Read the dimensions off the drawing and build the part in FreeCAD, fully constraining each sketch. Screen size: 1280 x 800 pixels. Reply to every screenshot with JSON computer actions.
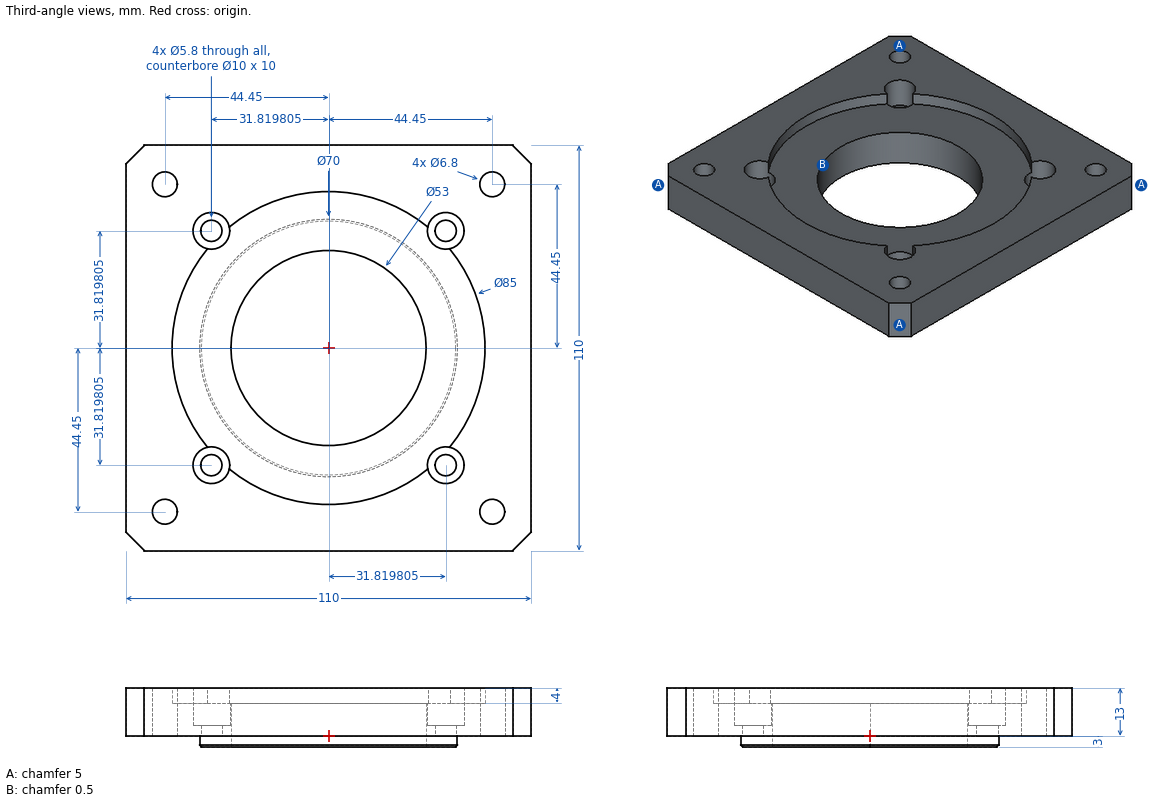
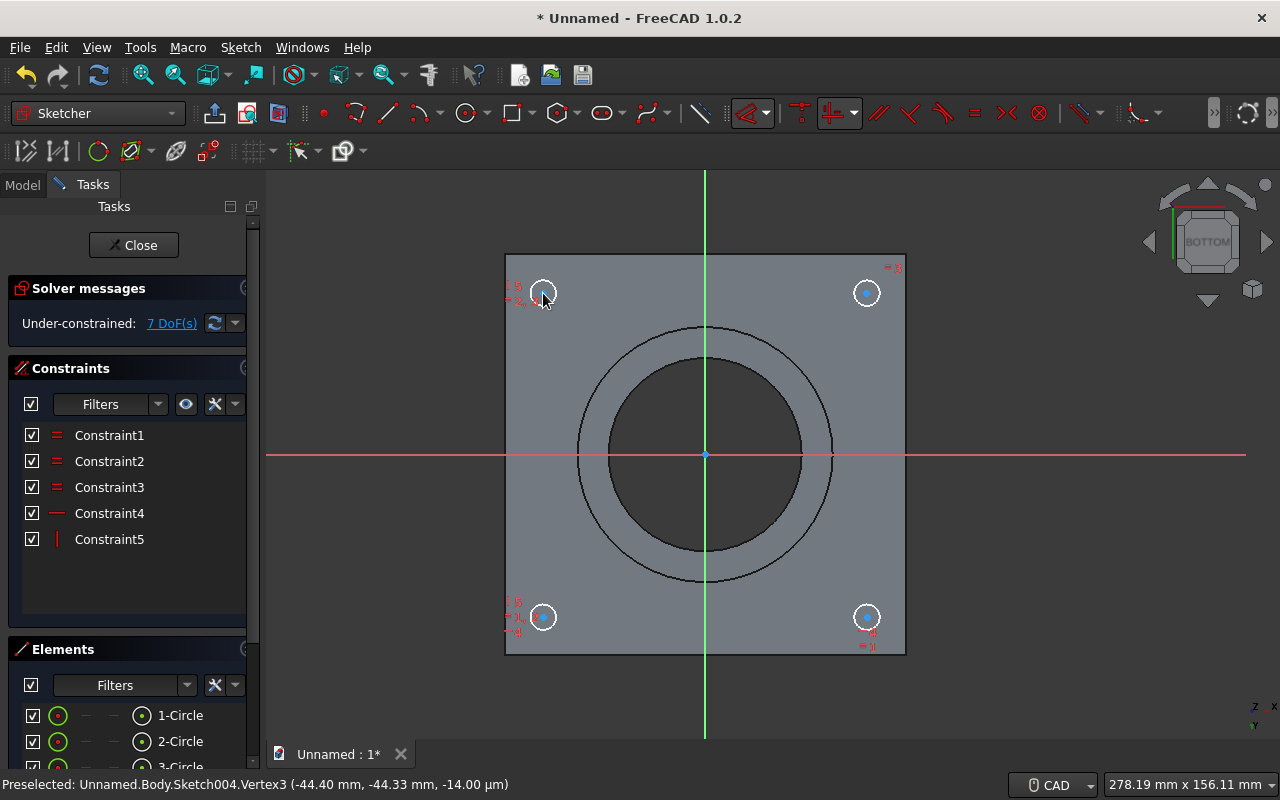
{"action": "left_click", "coordinate": [867, 617]}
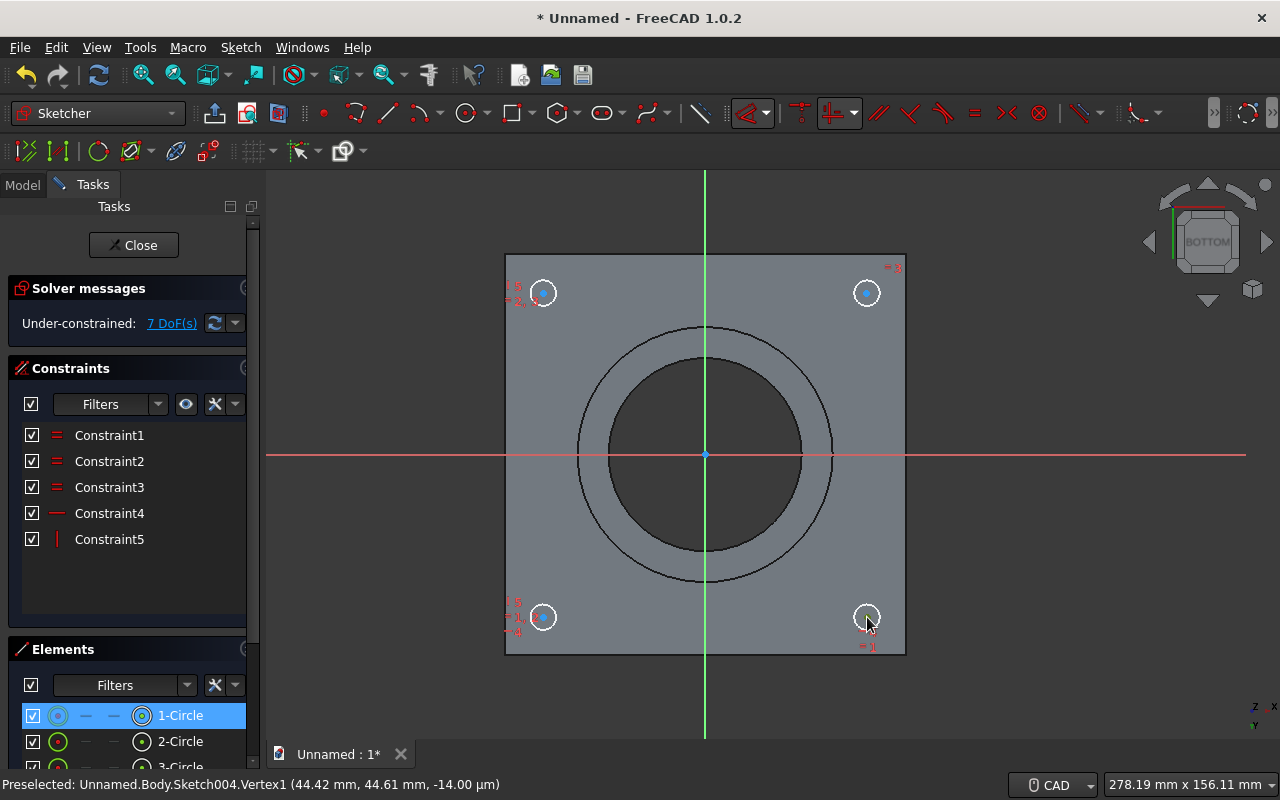
{"action": "left_click", "coordinate": [867, 293]}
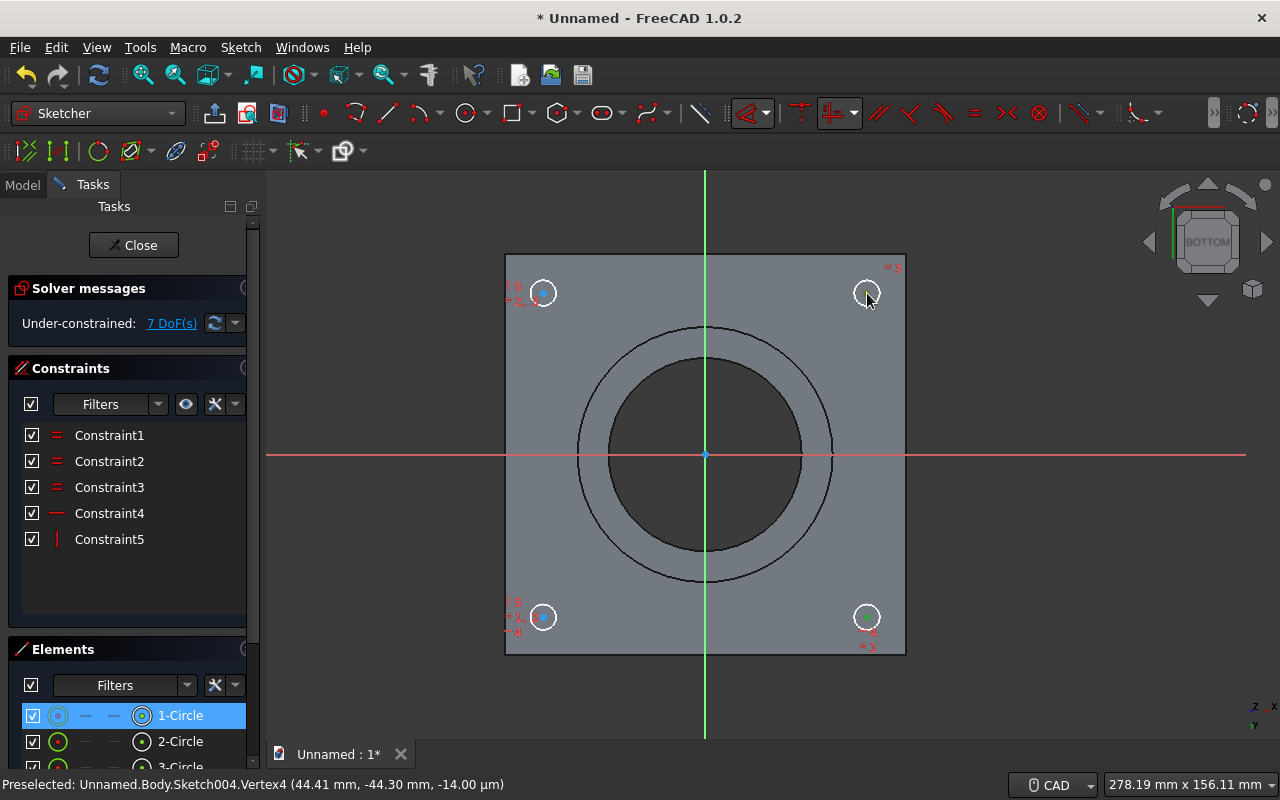
{"action": "key", "text": "v"}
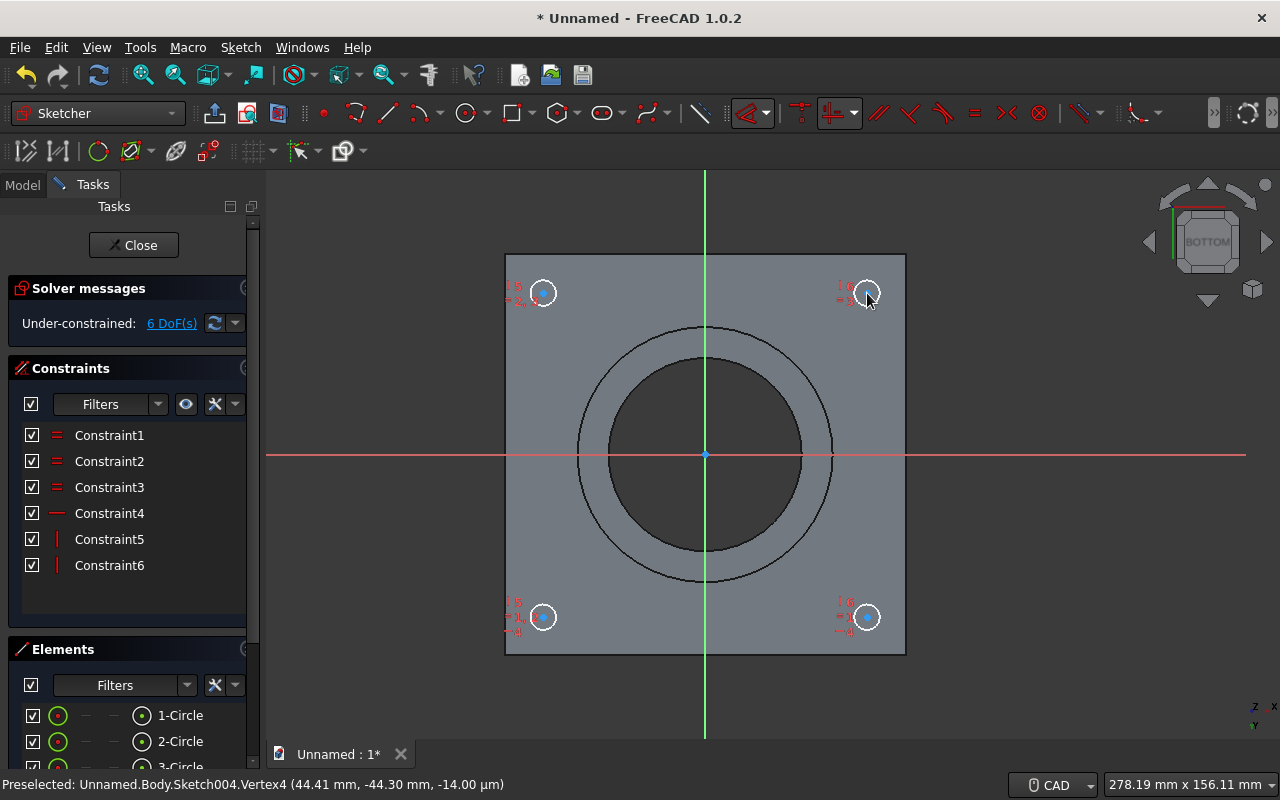
{"action": "left_click", "coordinate": [543, 293]}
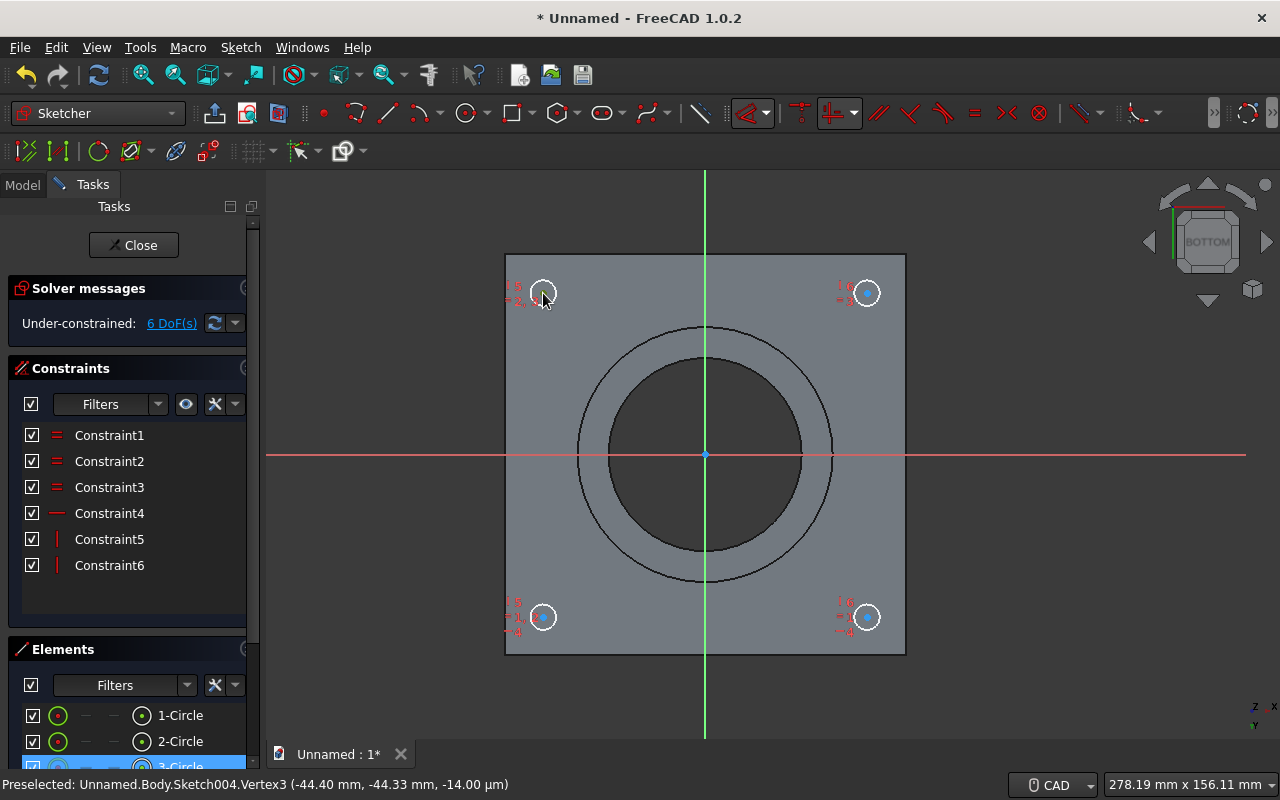
{"action": "left_click", "coordinate": [867, 293]}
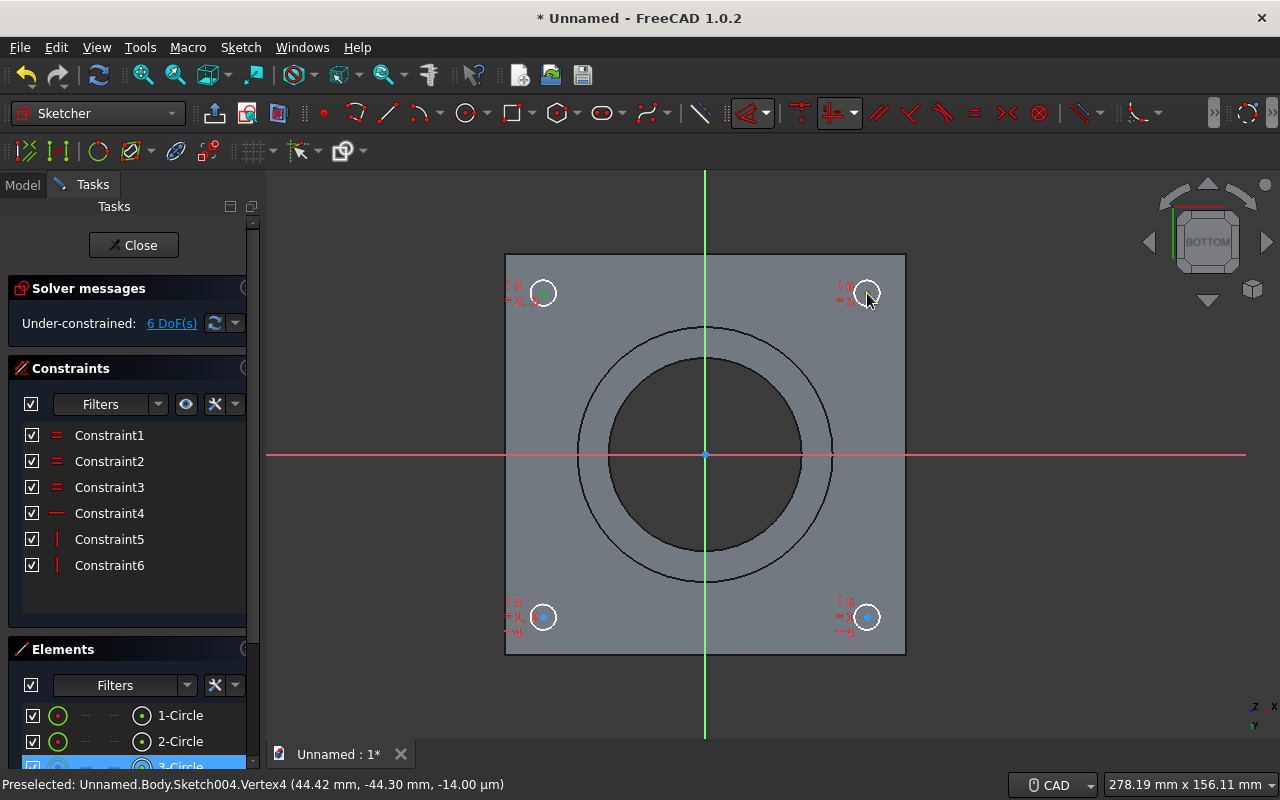
{"action": "key", "text": "h"}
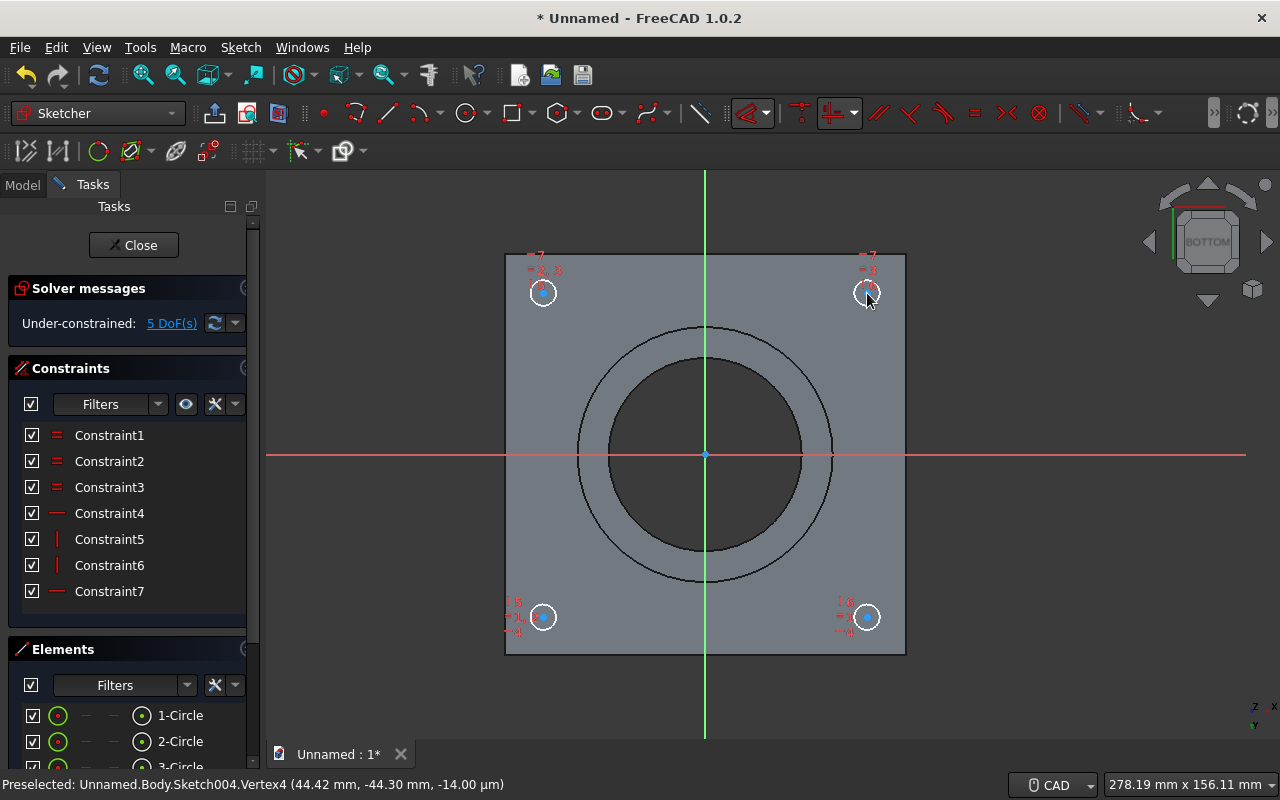
{"action": "scroll", "coordinate": [876, 608], "scroll_direction": "up", "scroll_amount": 3}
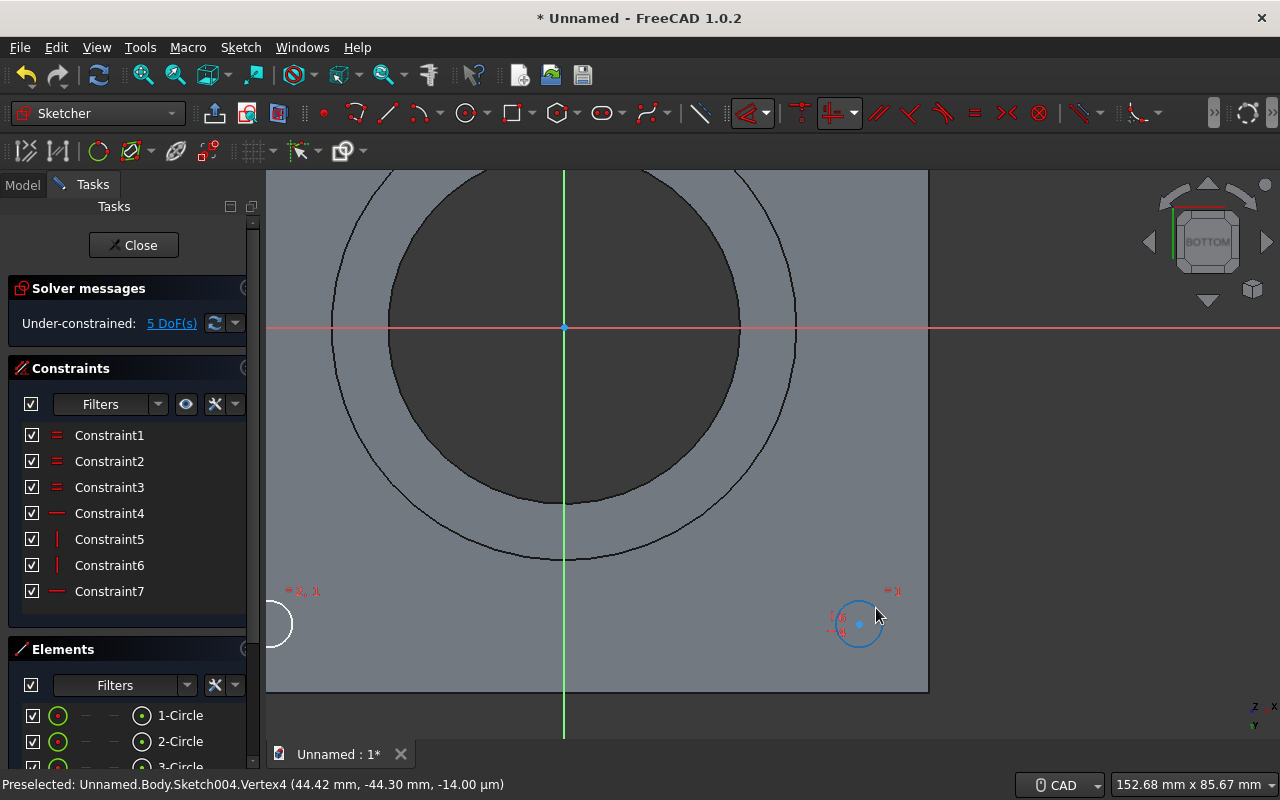
{"action": "left_click", "coordinate": [875, 608]}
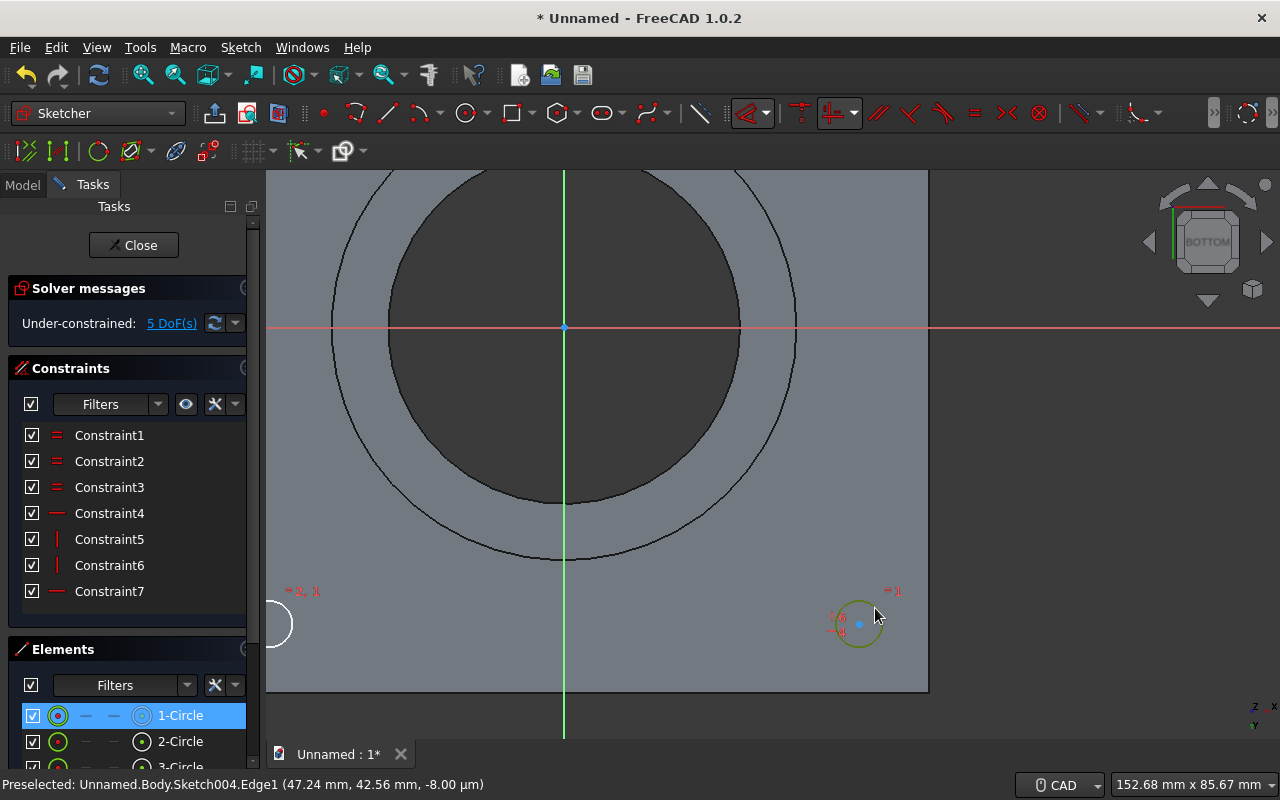
{"action": "key", "text": "k o"}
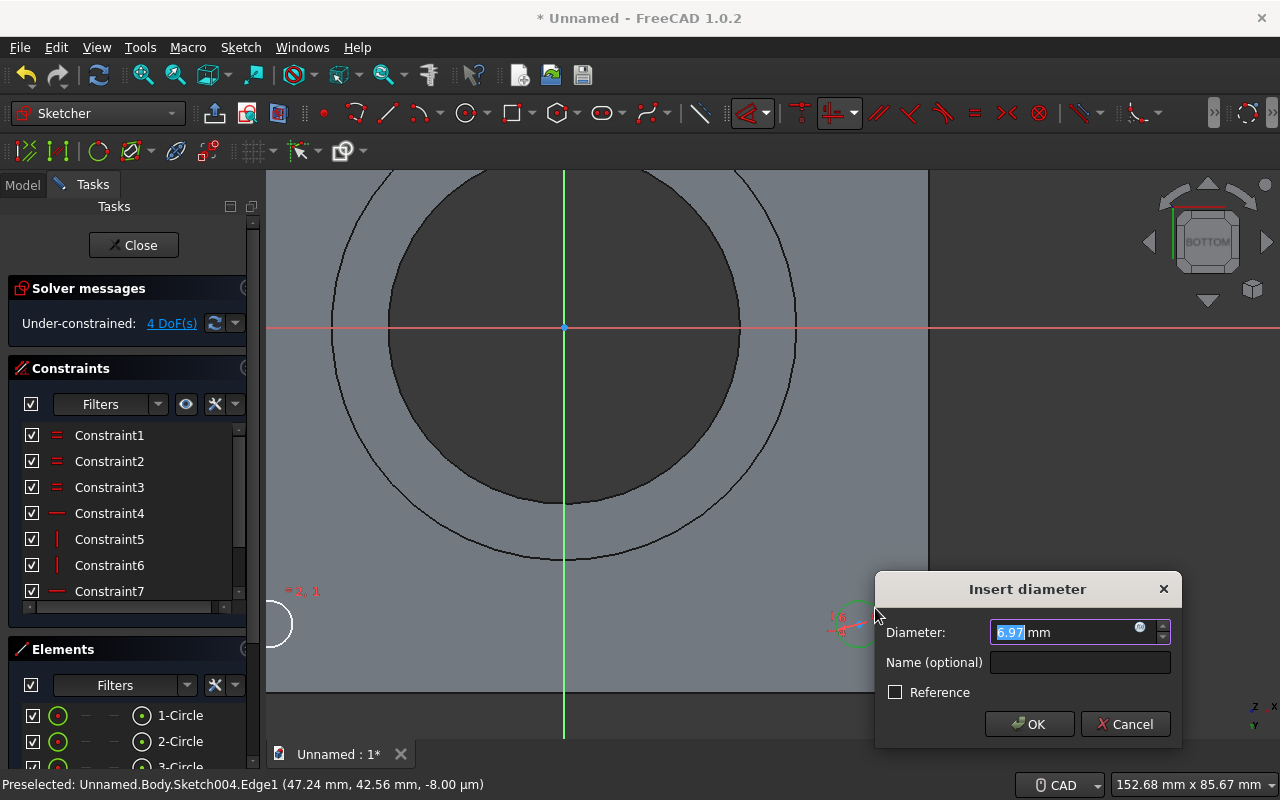
{"action": "type", "text": "6.8"}
{"action": "key", "text": "Return"}